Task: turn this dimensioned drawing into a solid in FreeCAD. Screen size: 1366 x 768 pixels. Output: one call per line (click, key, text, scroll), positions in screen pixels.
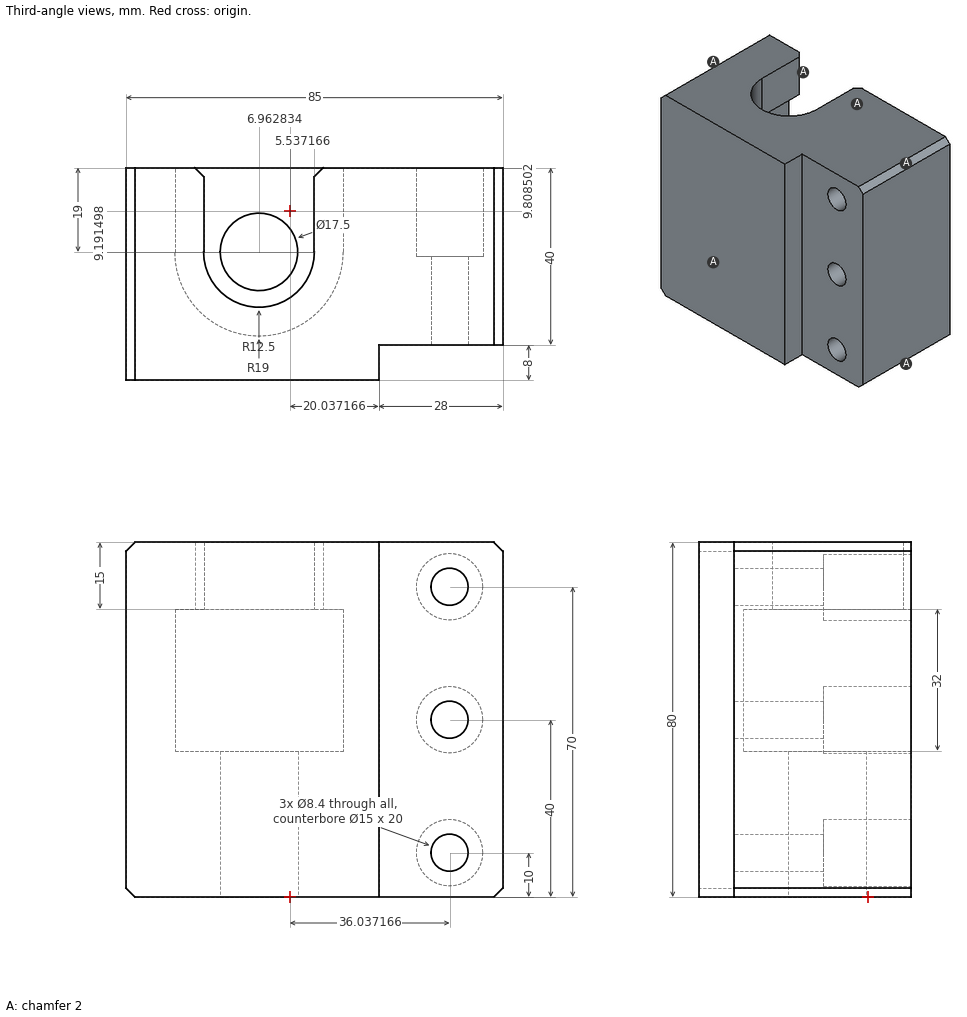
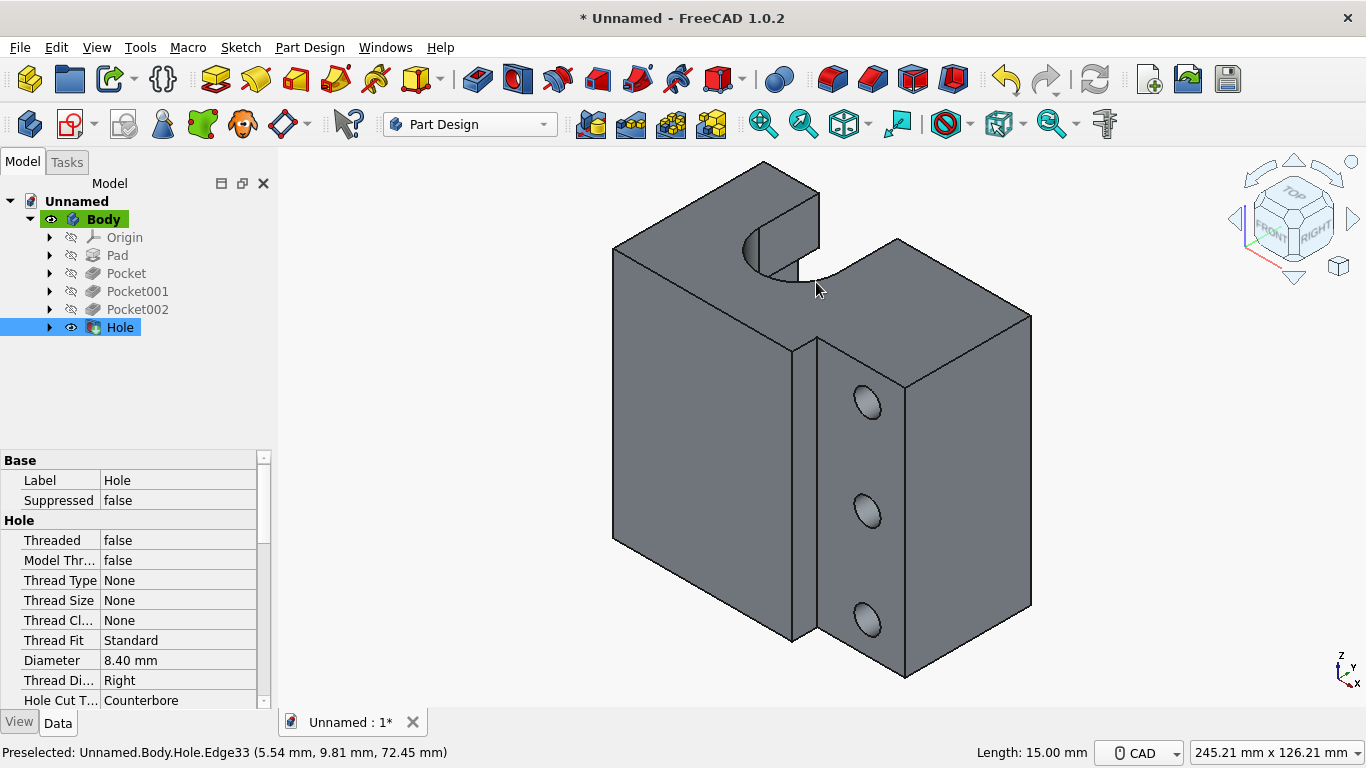
click(968, 351, ctrl)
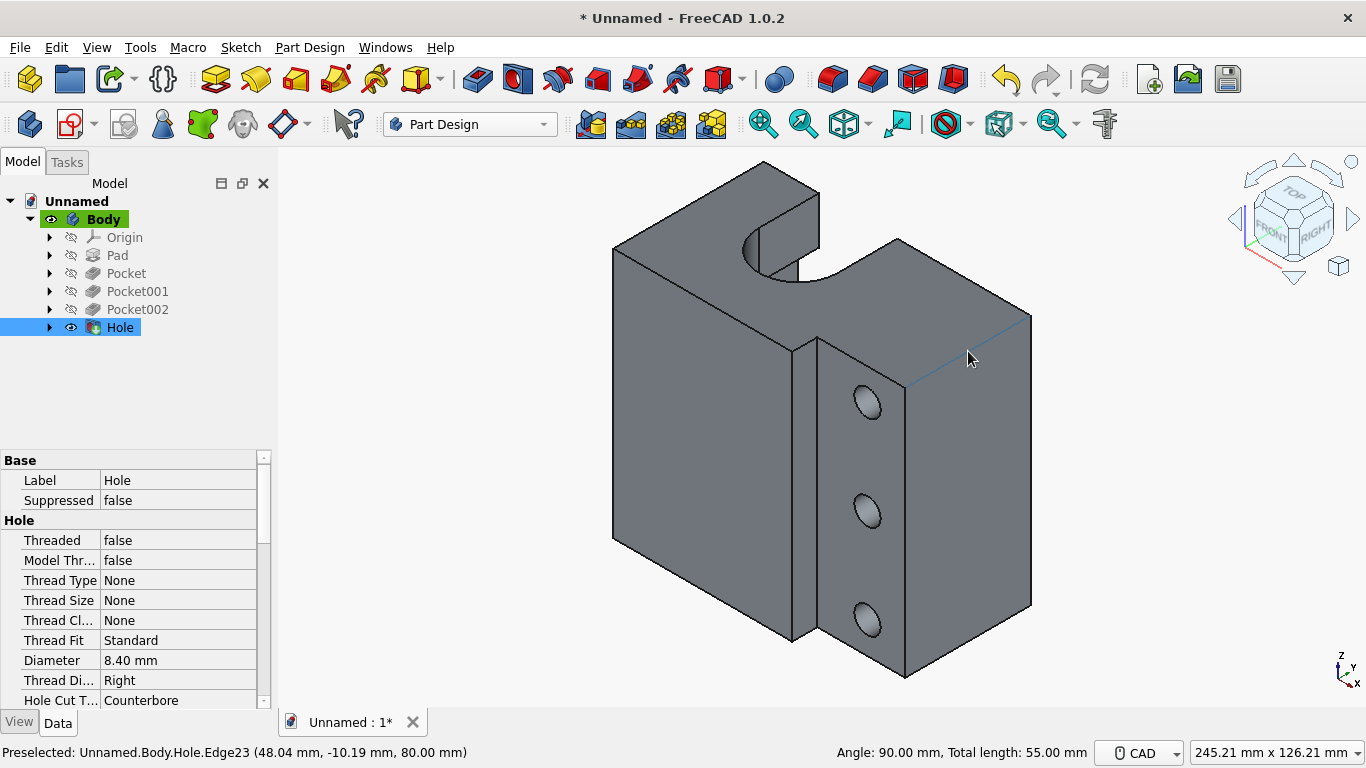
key(2)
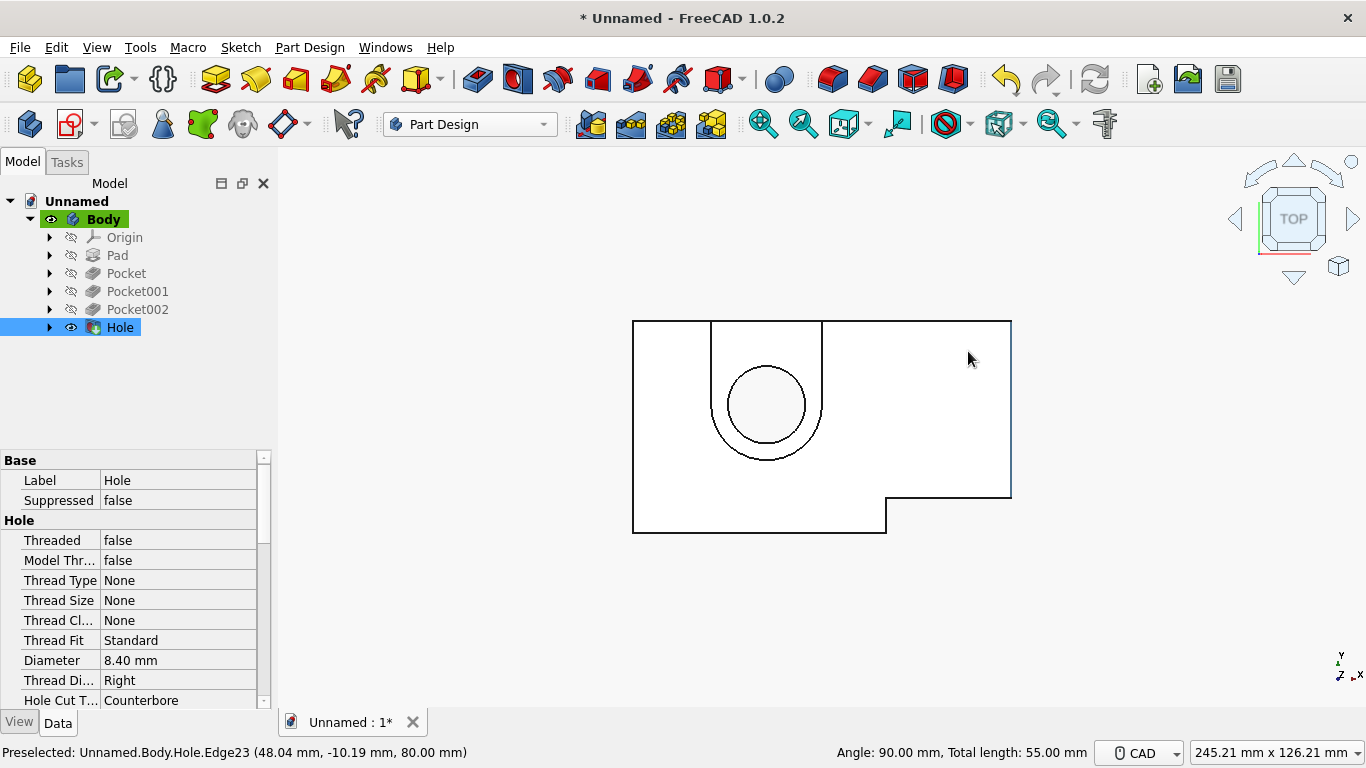
click(764, 124)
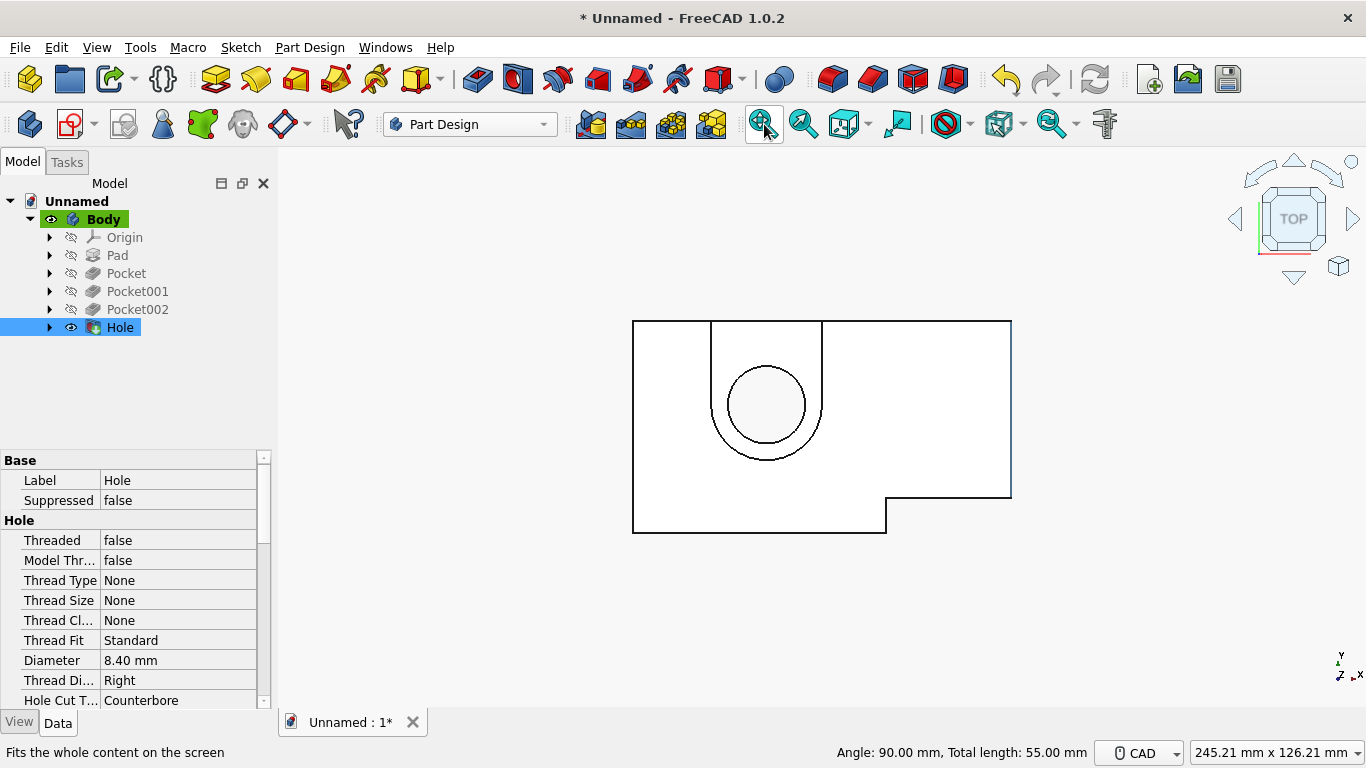
click(633, 426, ctrl)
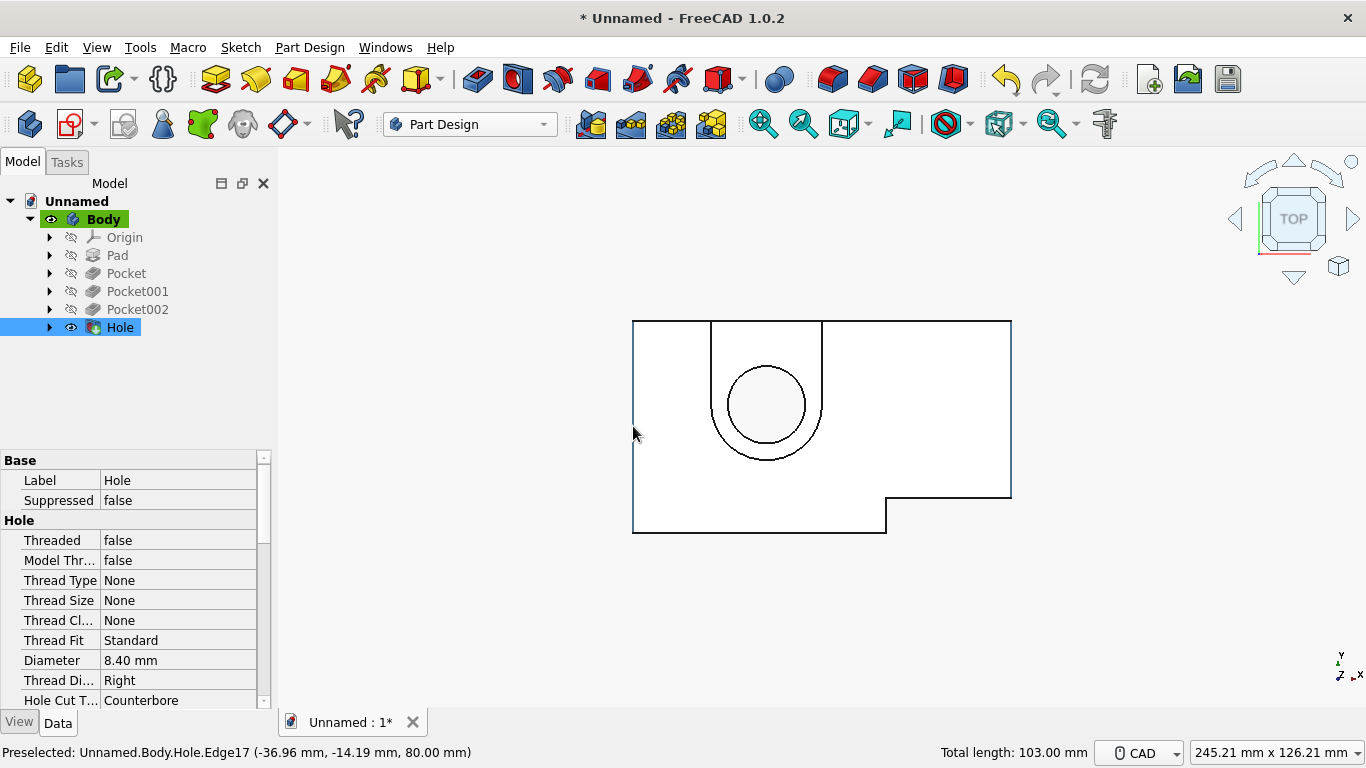
key(1)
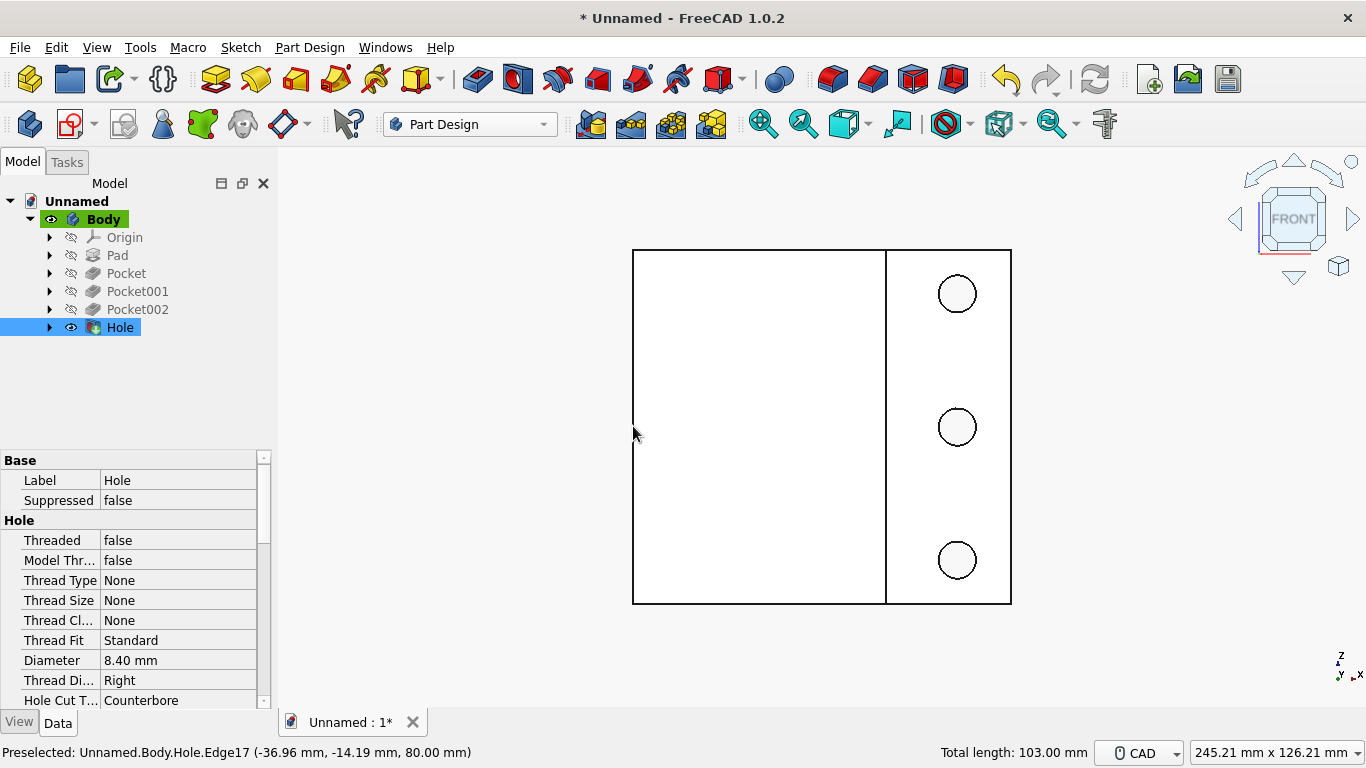
key(3)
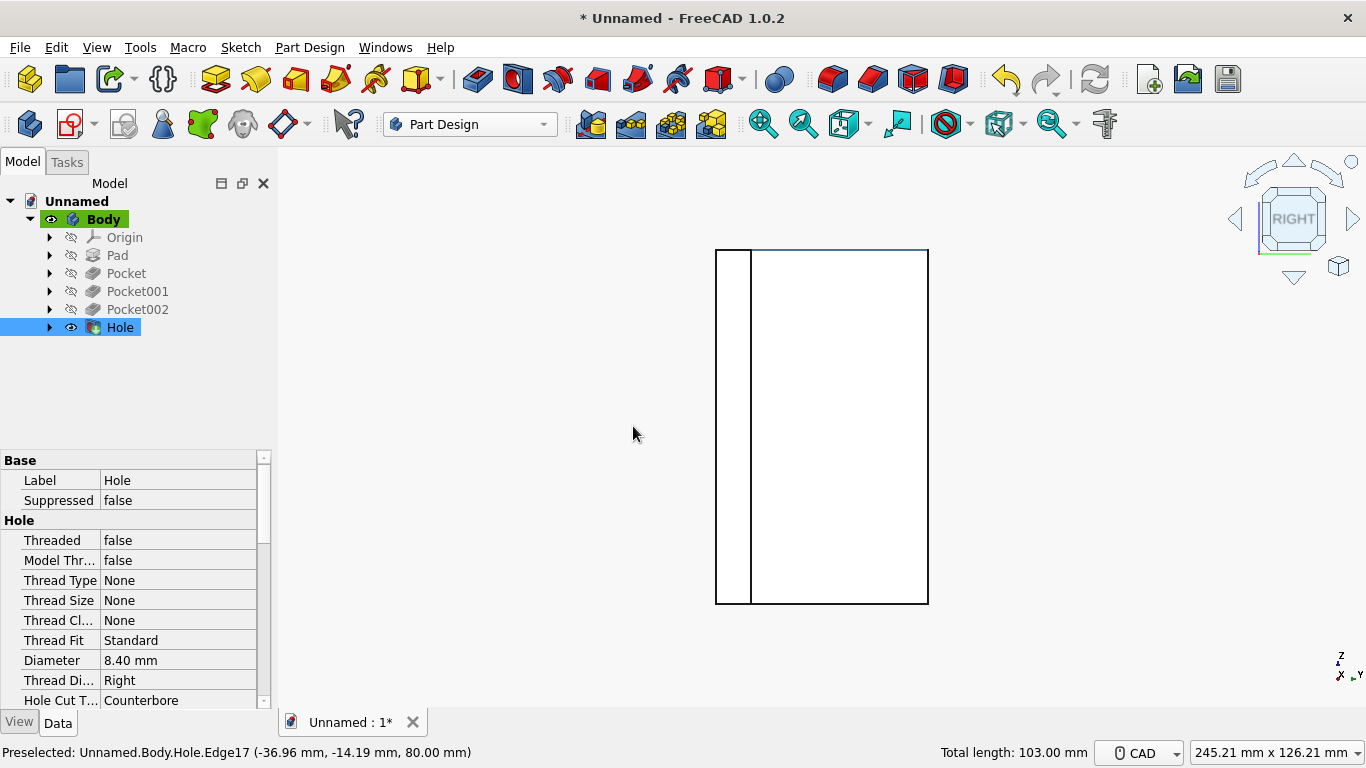
click(840, 603, ctrl)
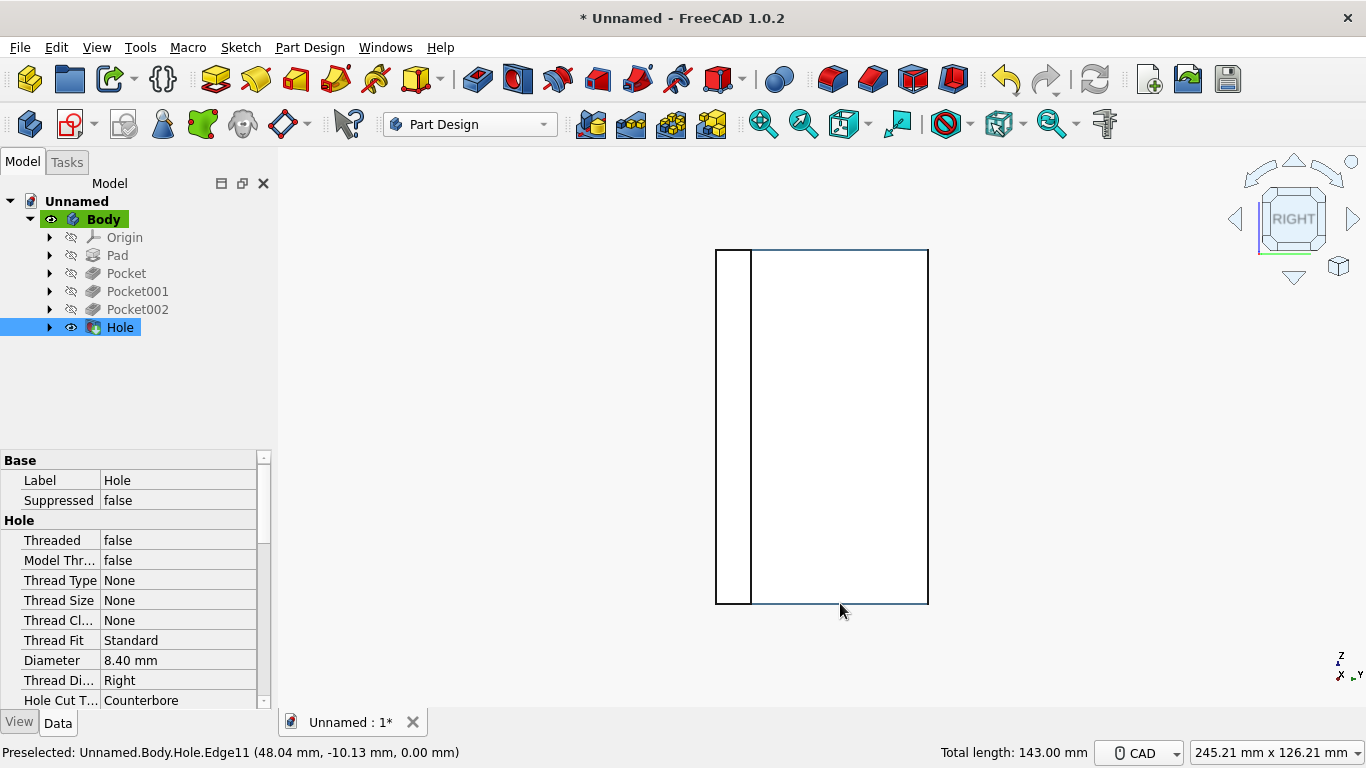
key(5)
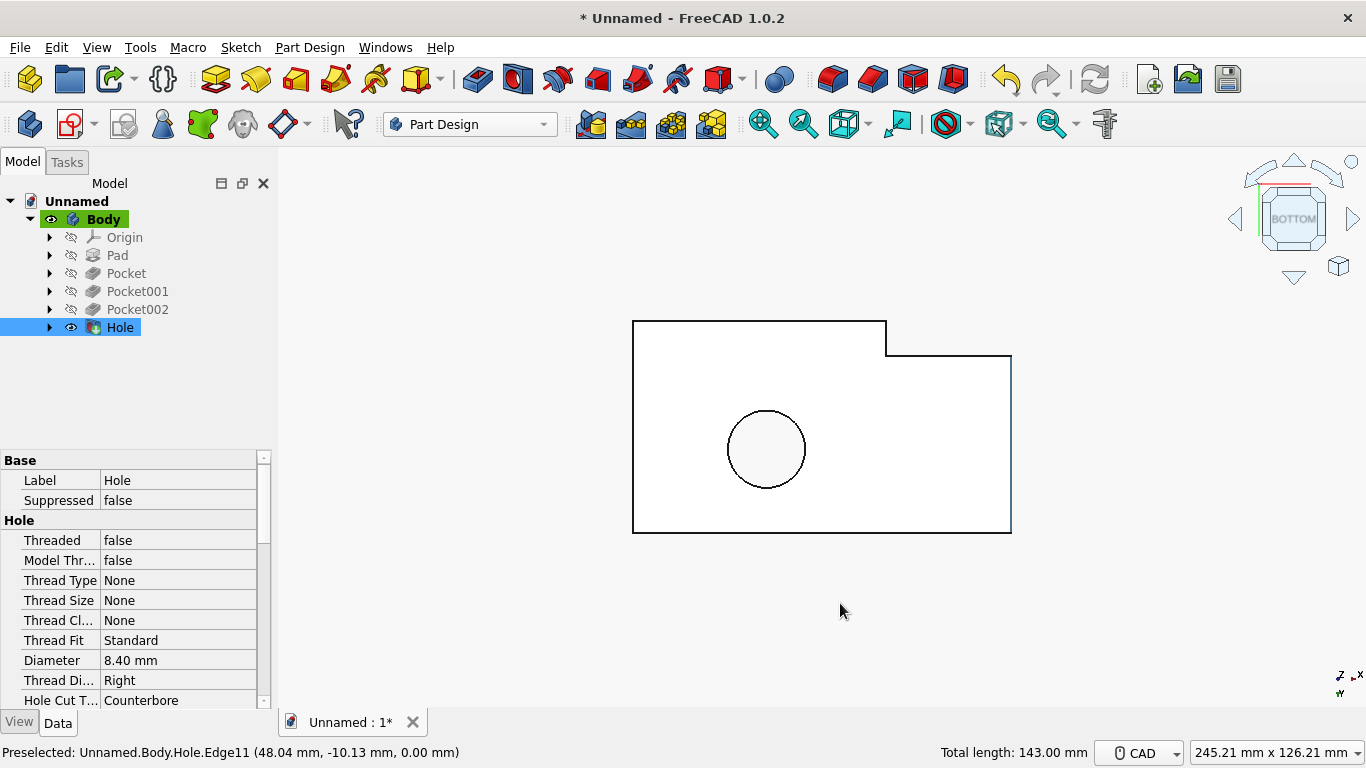
click(764, 124)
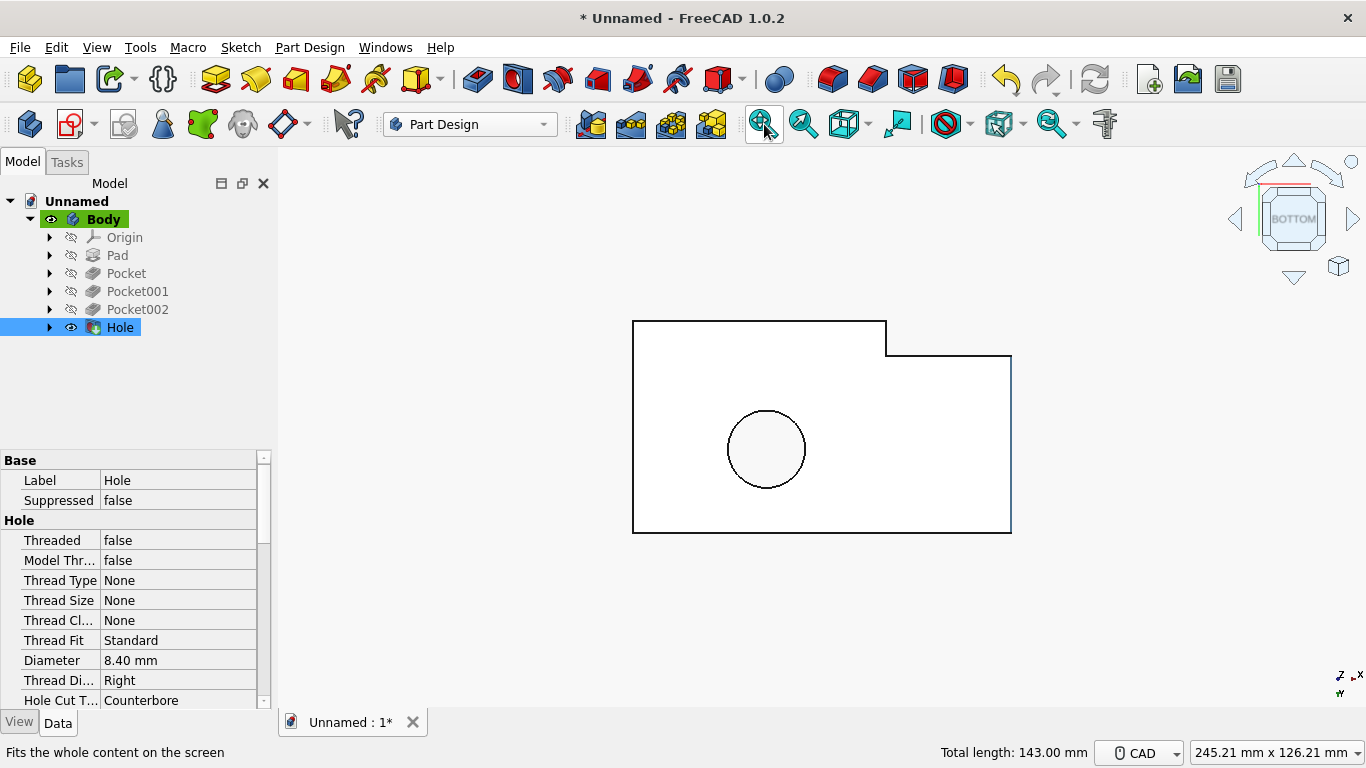
click(633, 426, ctrl)